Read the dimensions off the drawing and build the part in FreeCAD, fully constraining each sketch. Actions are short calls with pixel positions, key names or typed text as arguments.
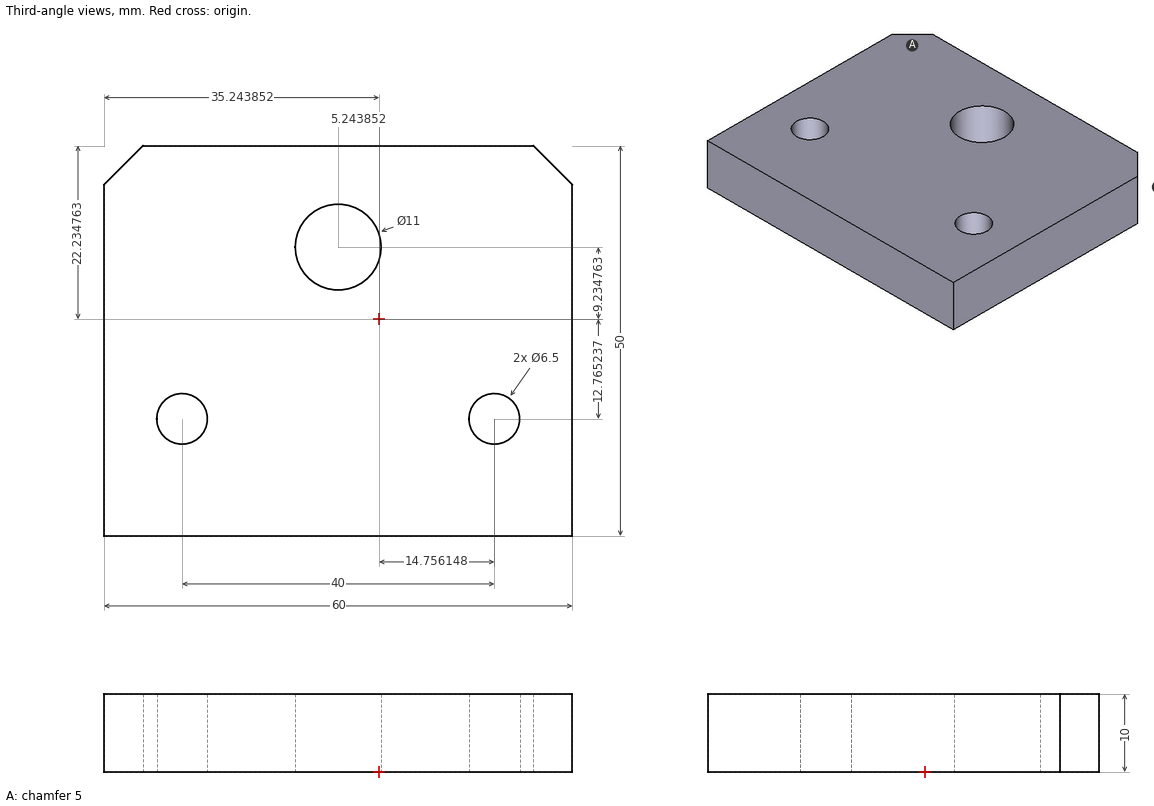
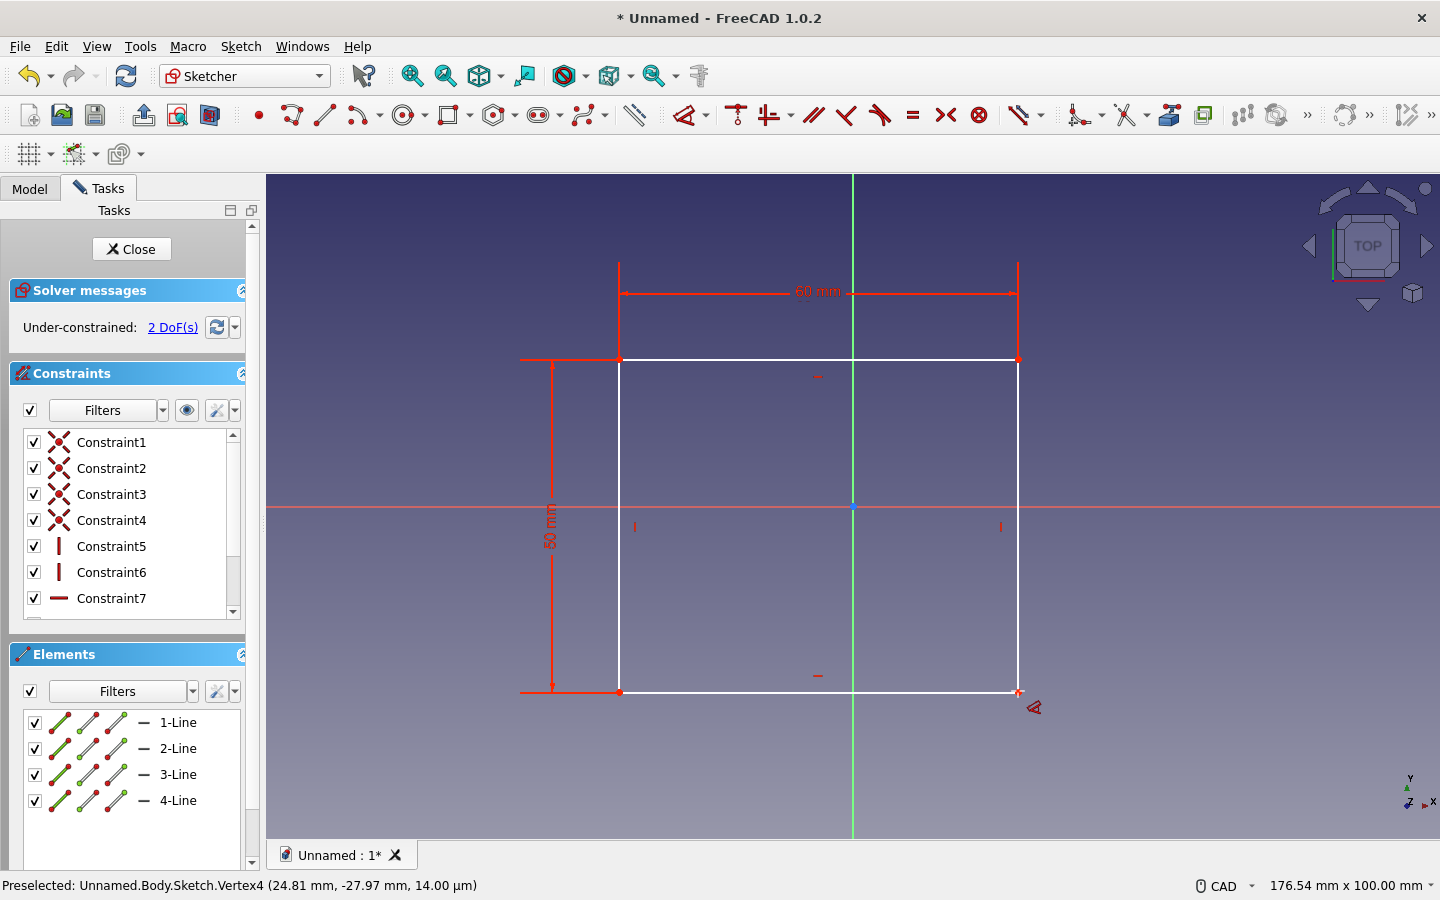
click(619, 360)
click(736, 326)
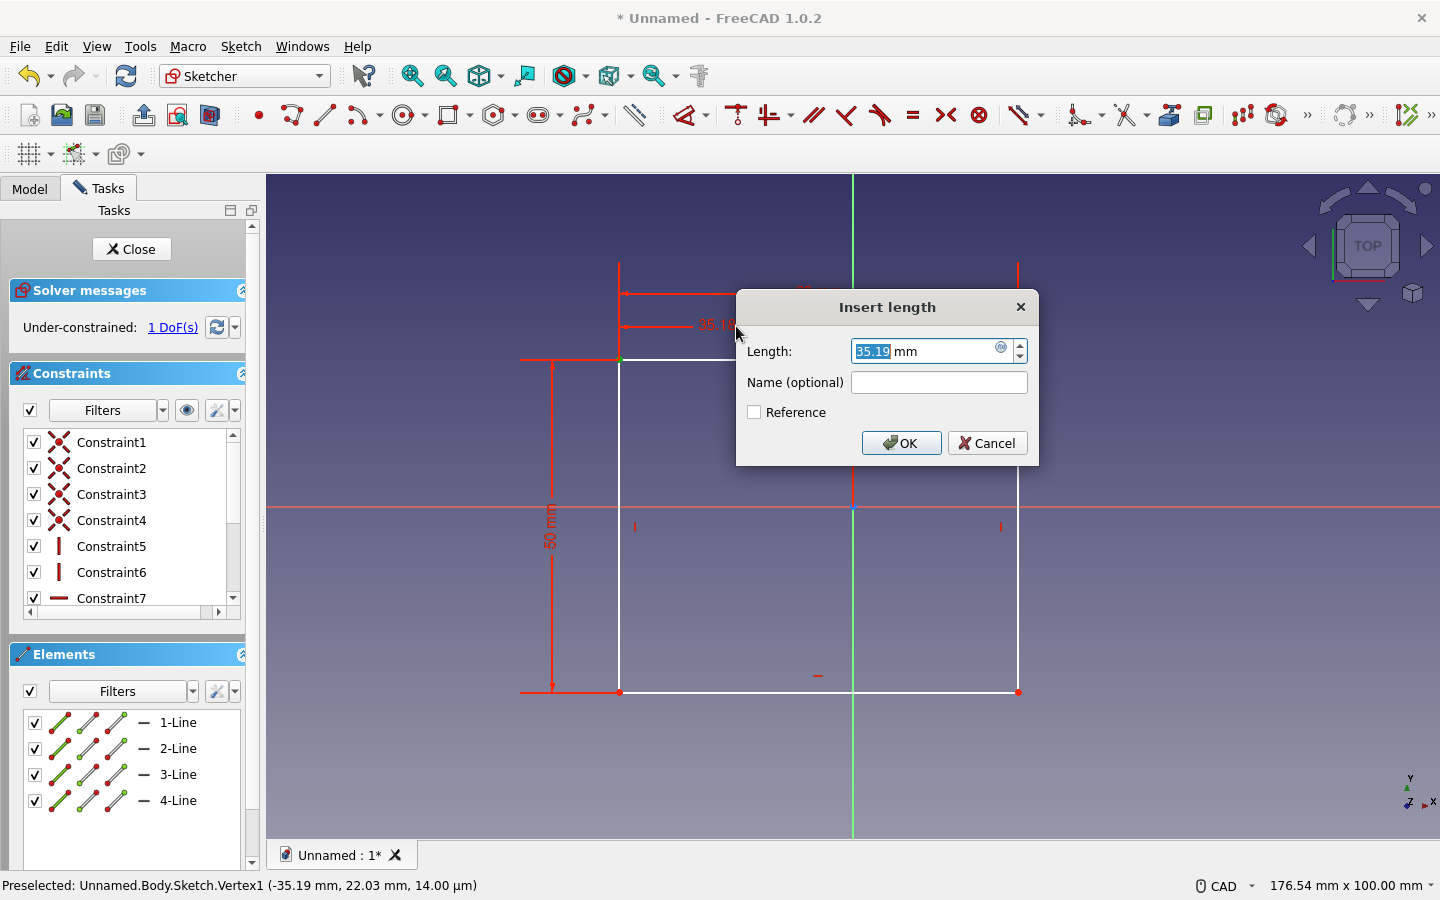
text(35.243852)
key(Return)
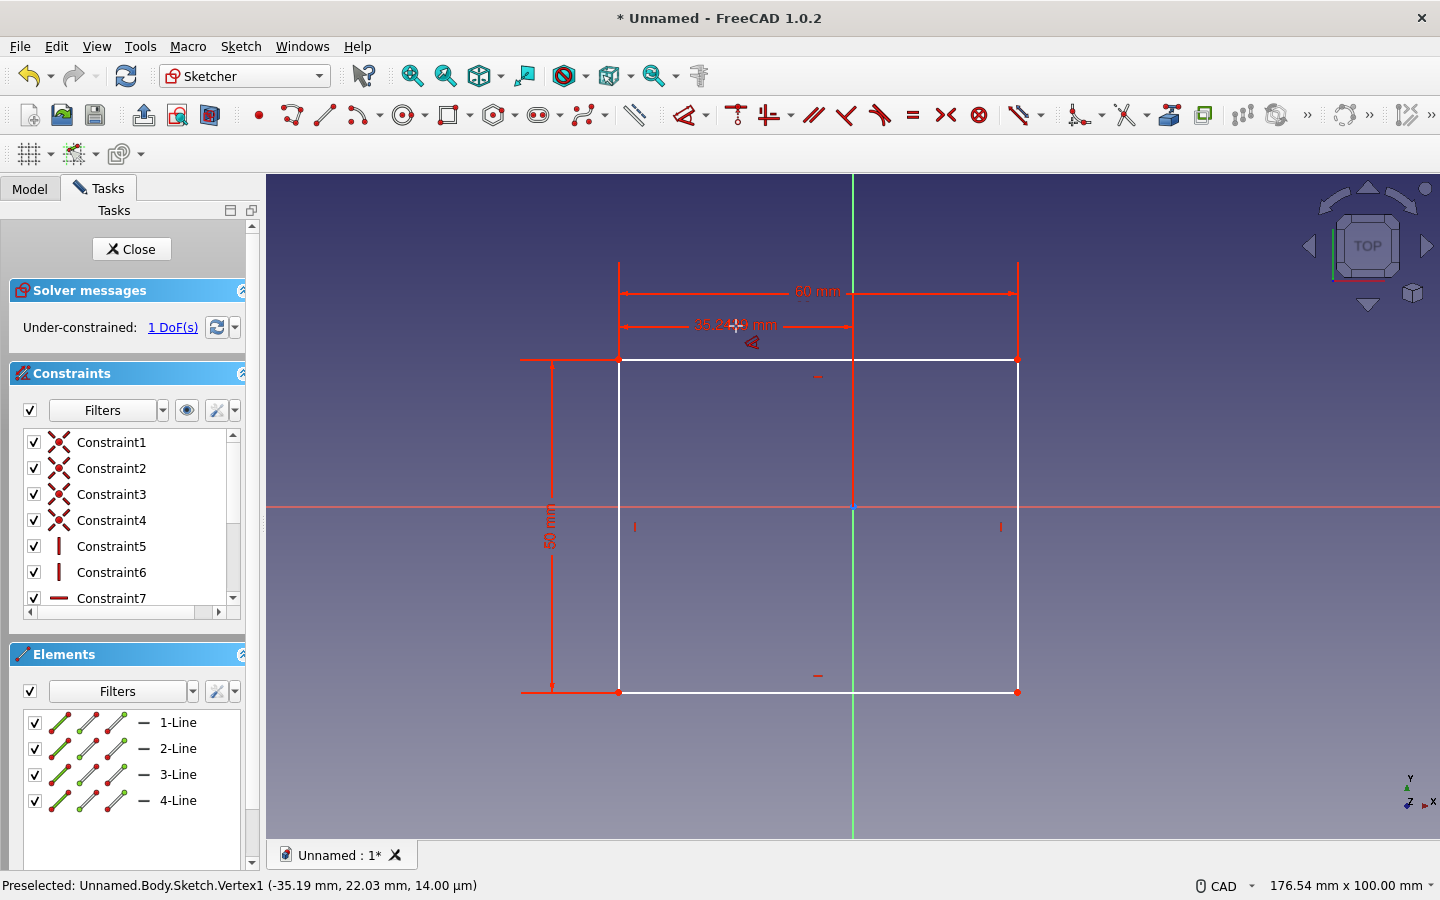
click(619, 360)
click(585, 433)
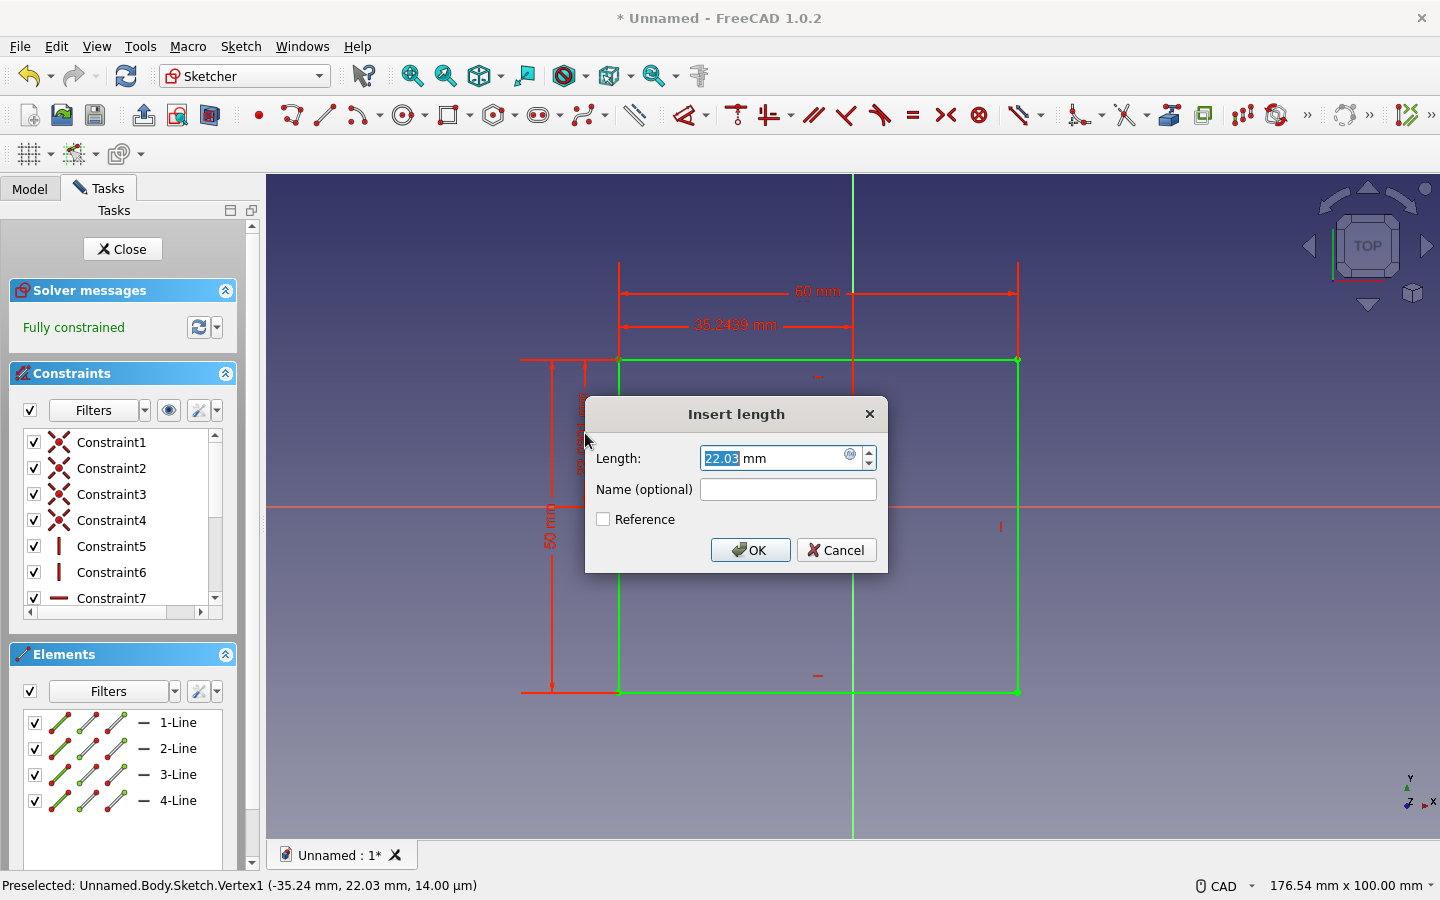
text(22.234763)
key(Return)
key(Escape)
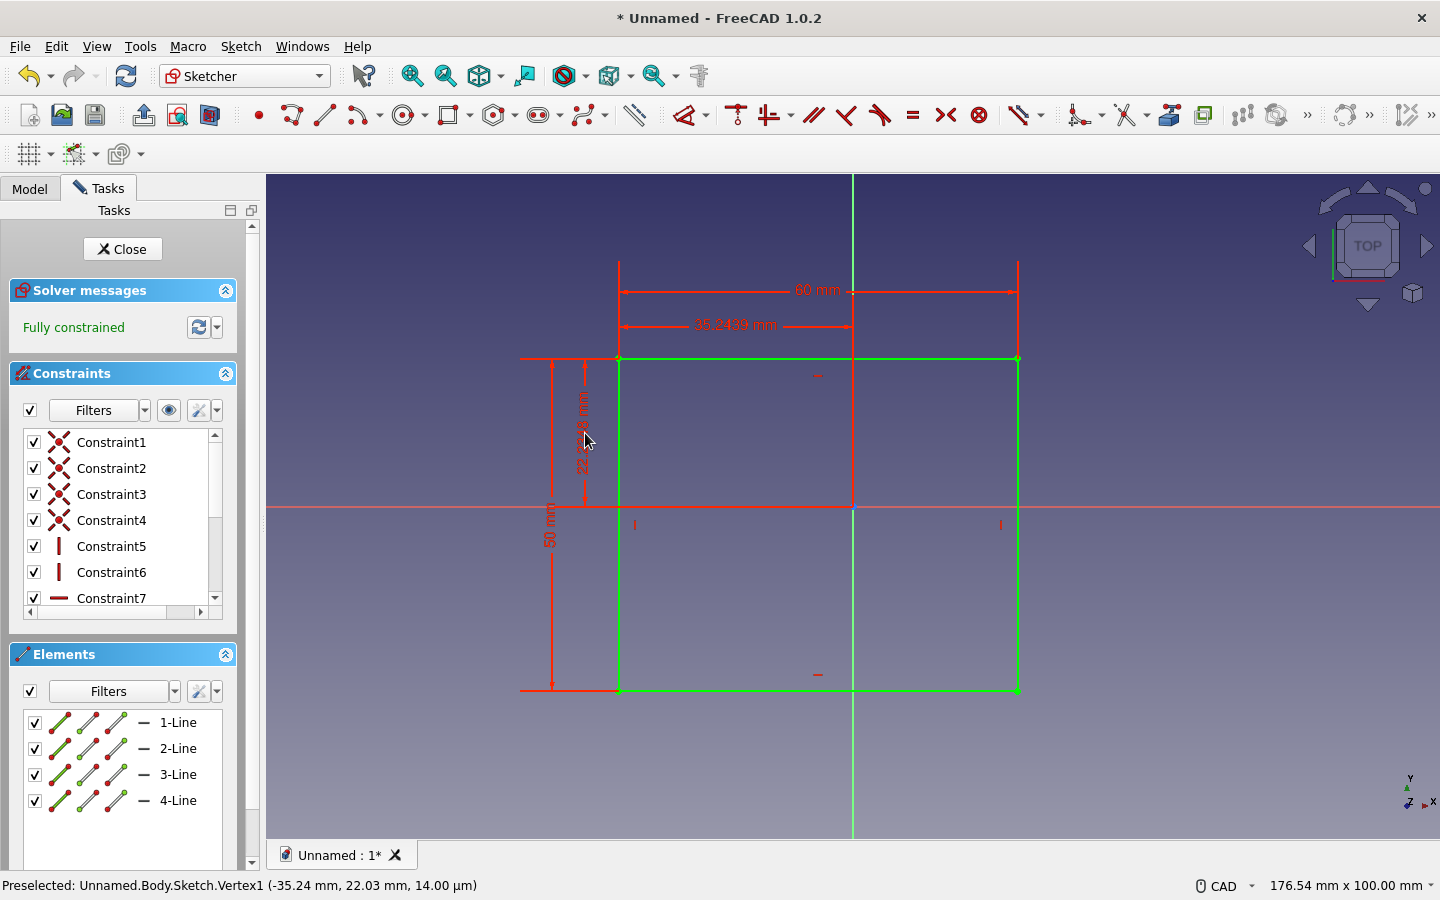
click(123, 249)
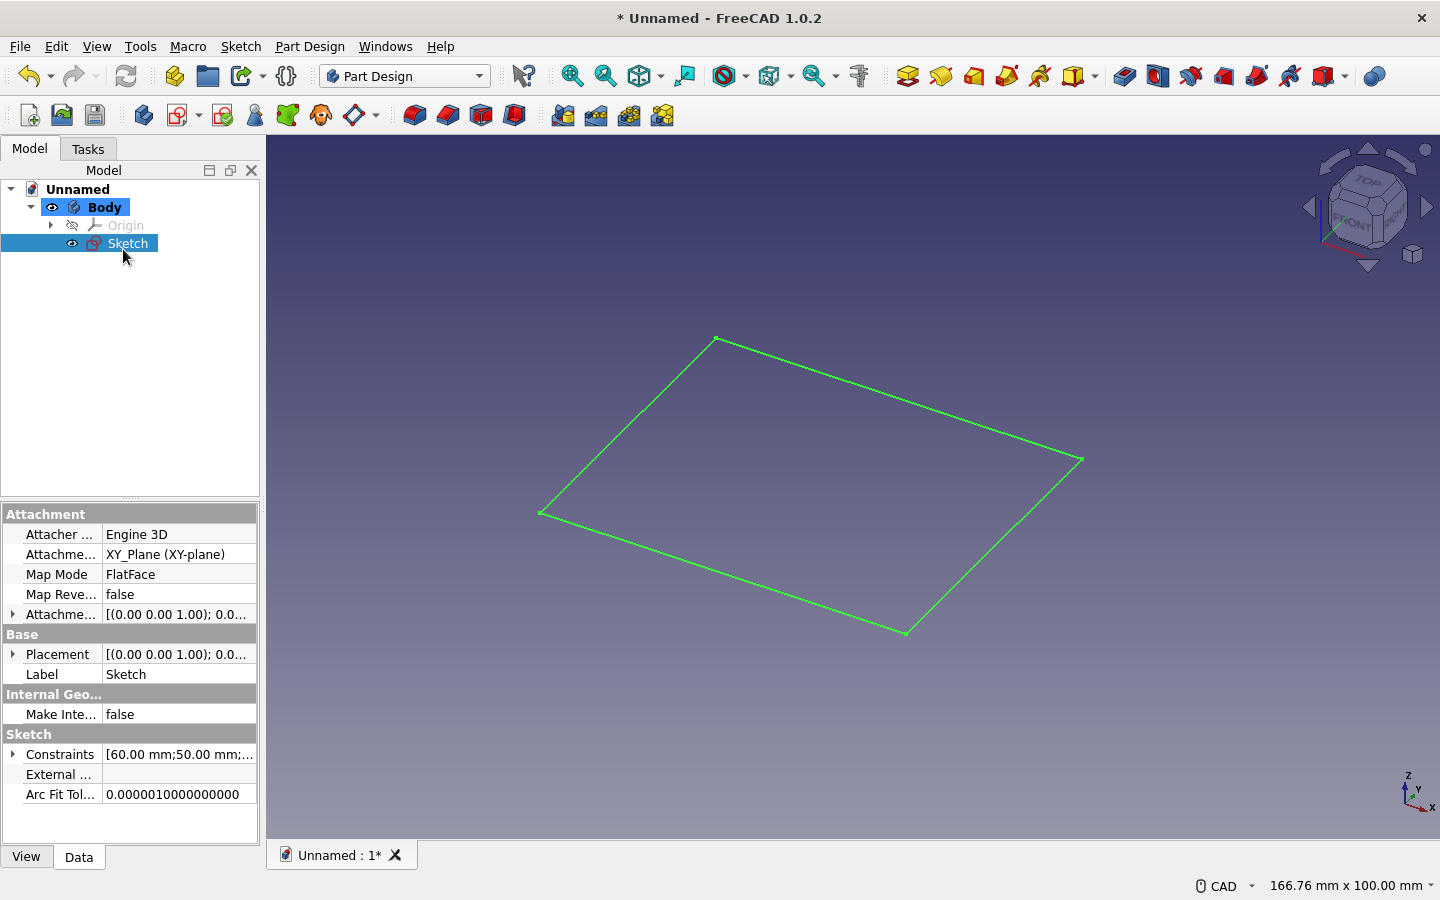
click(908, 76)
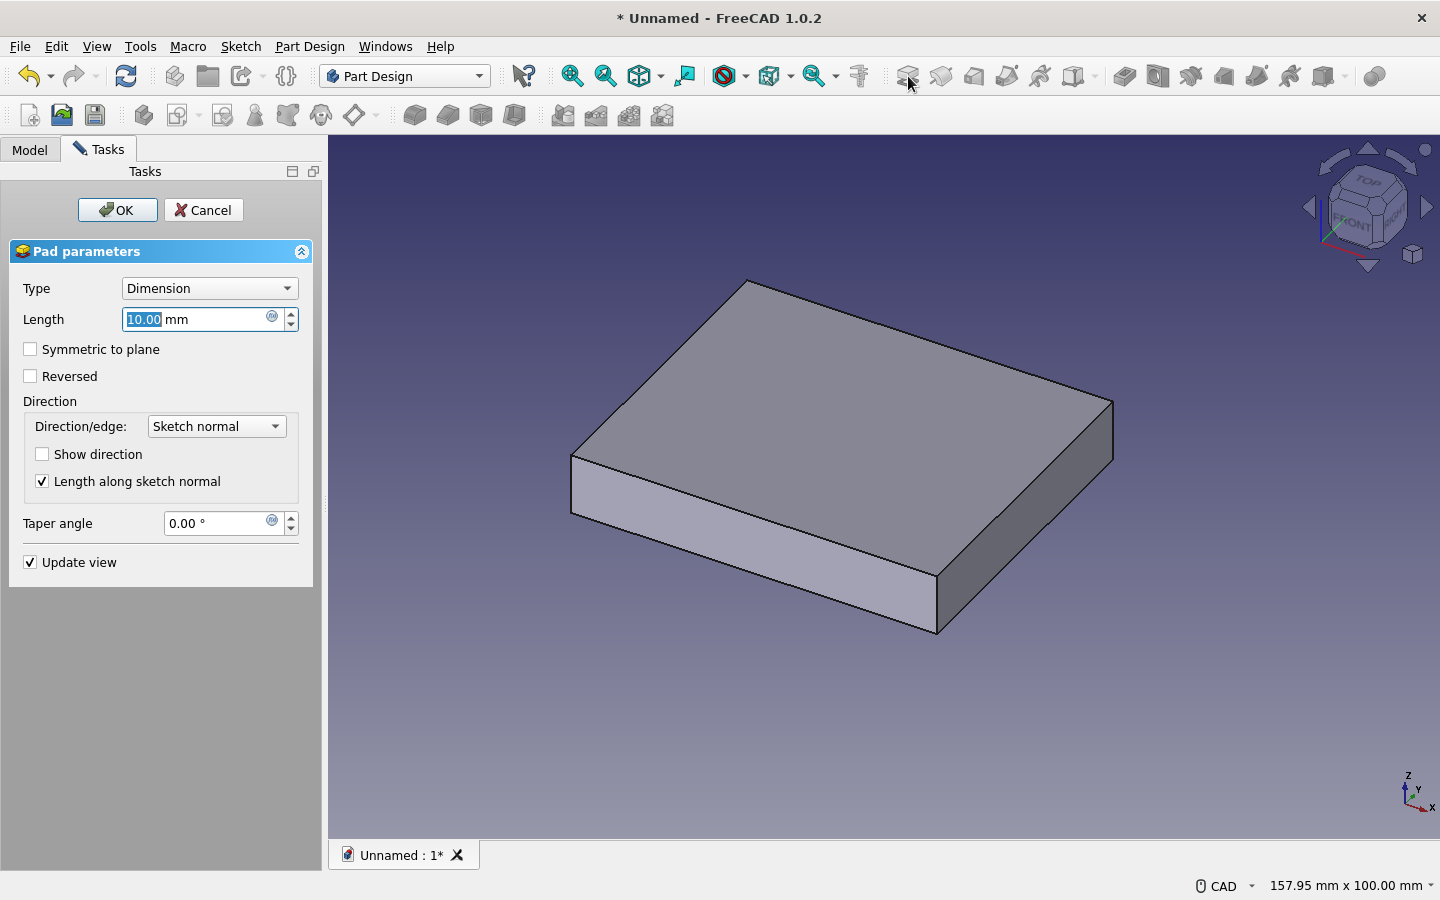
text(10)
key(Tab)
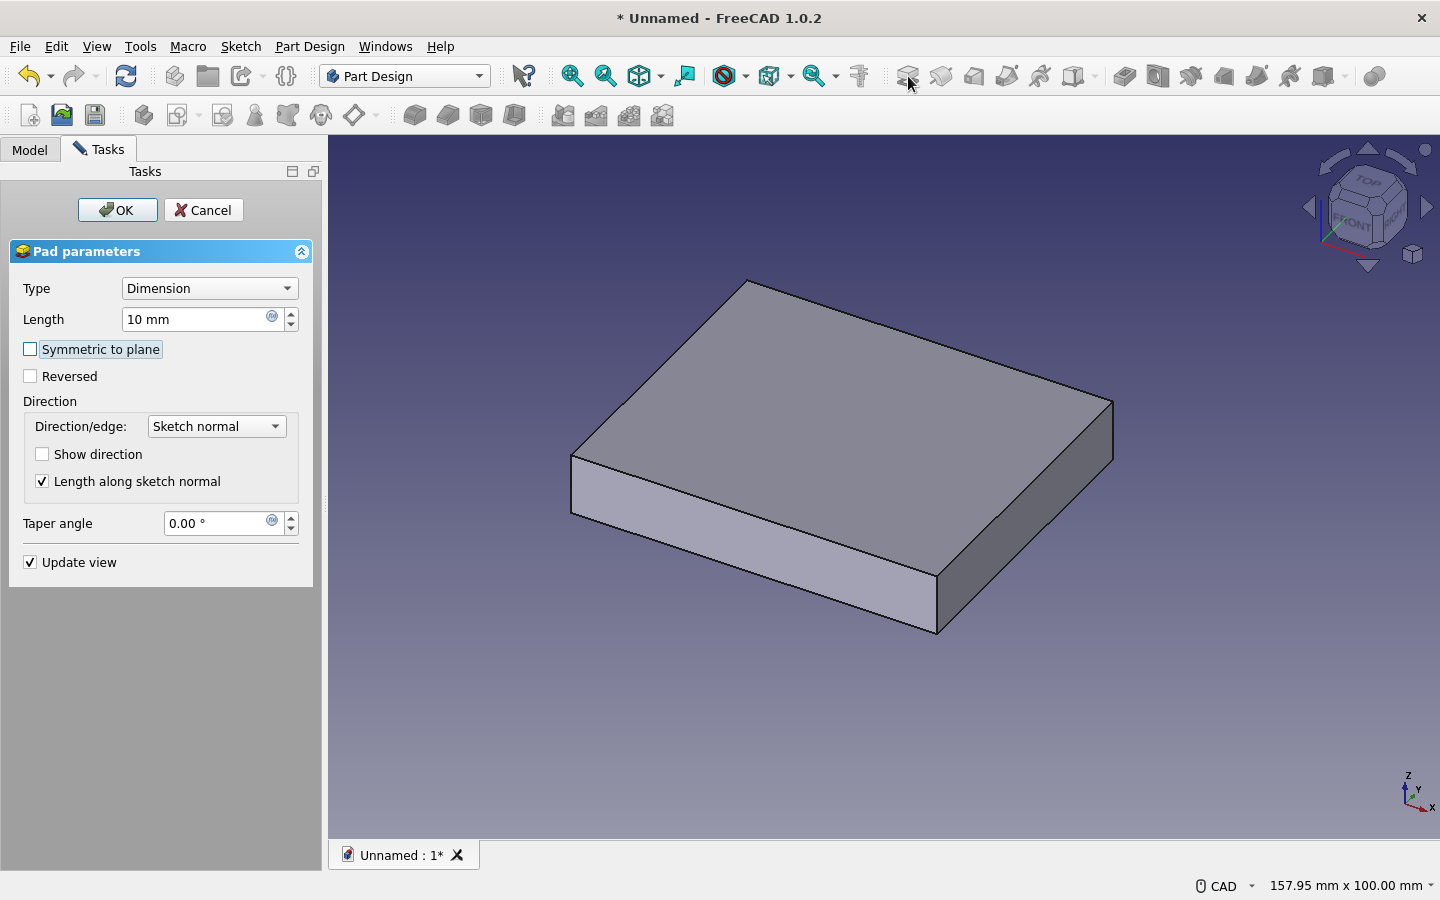
click(118, 210)